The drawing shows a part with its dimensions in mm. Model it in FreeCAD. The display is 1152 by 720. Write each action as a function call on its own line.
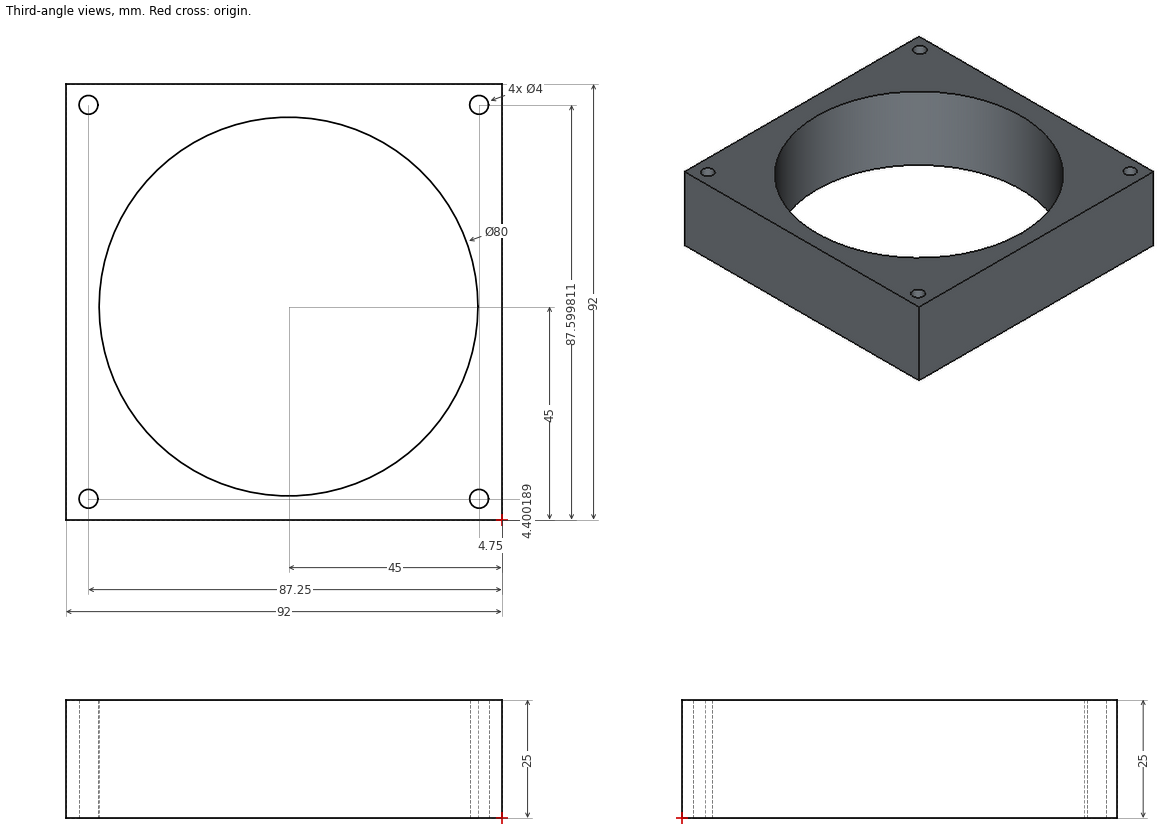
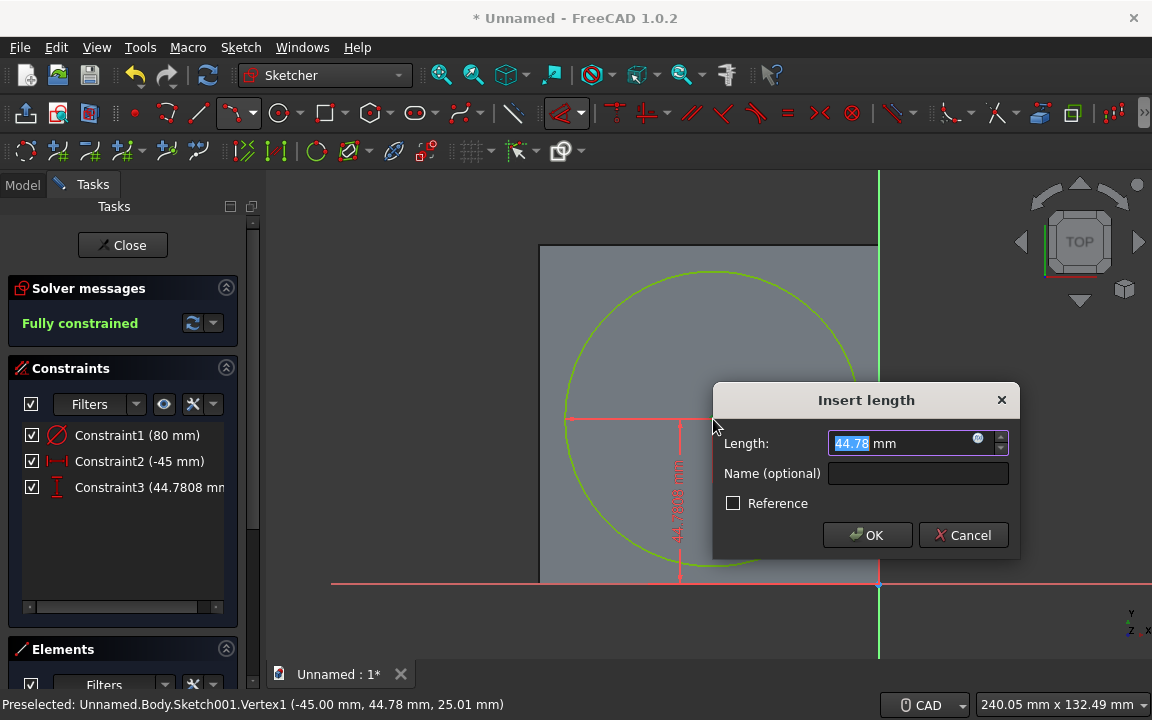
text(45)
key(Return)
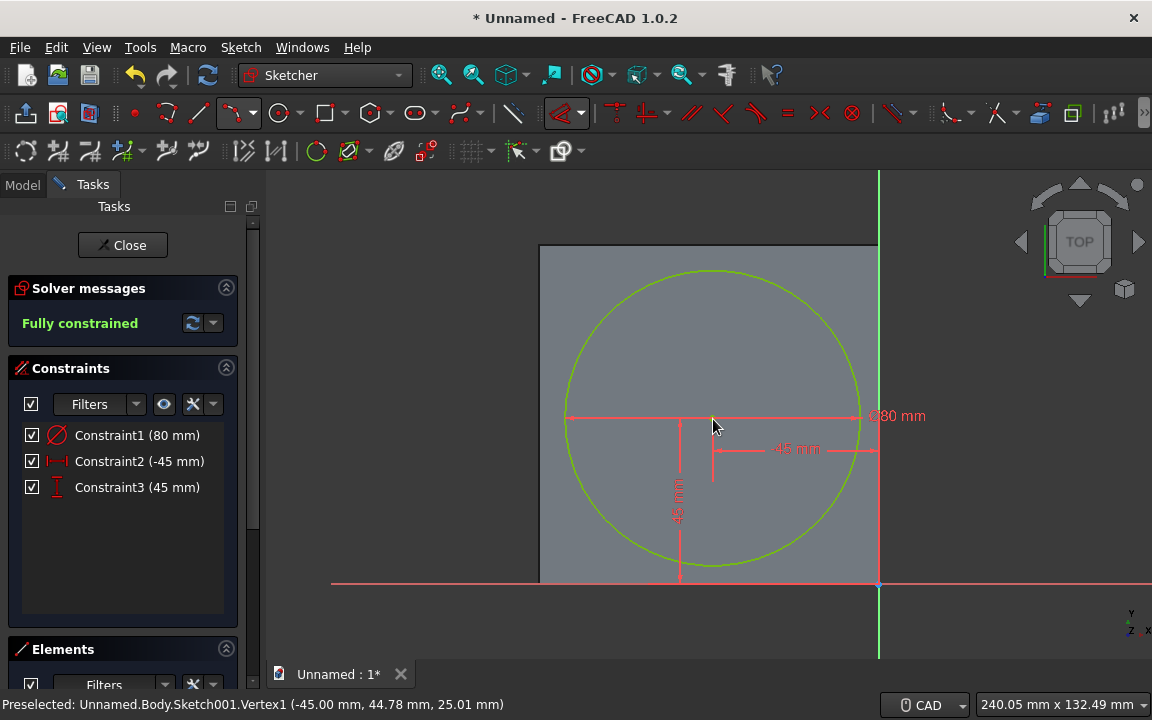
click(123, 245)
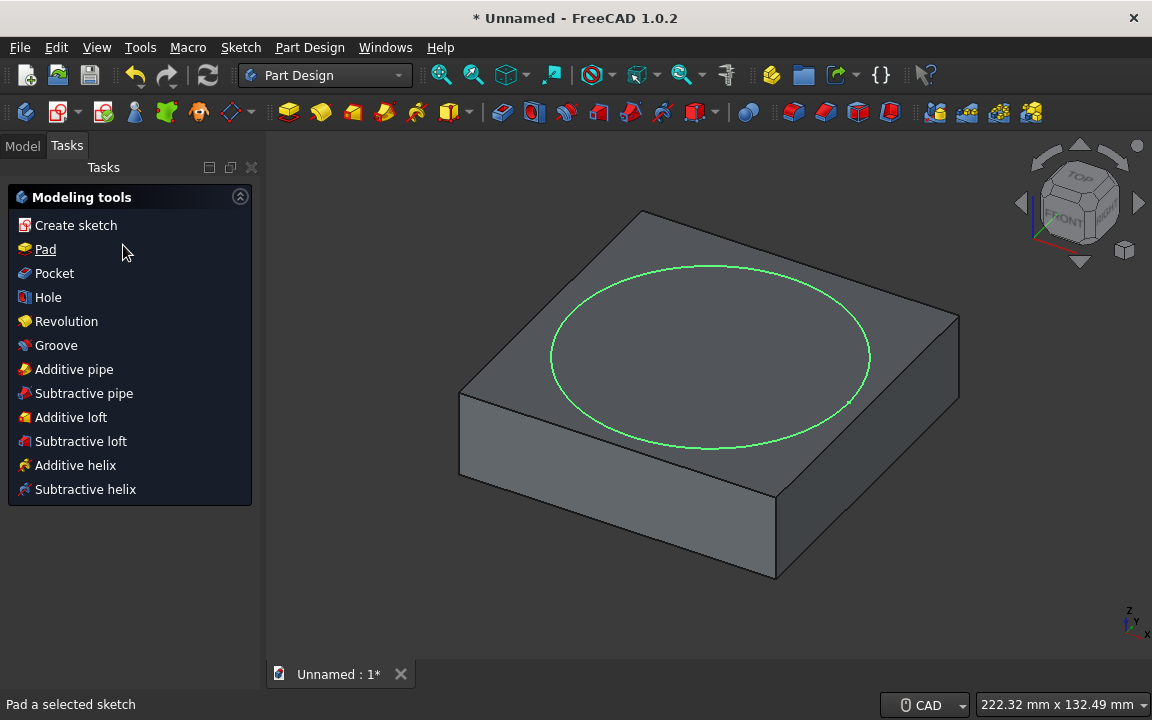
click(504, 112)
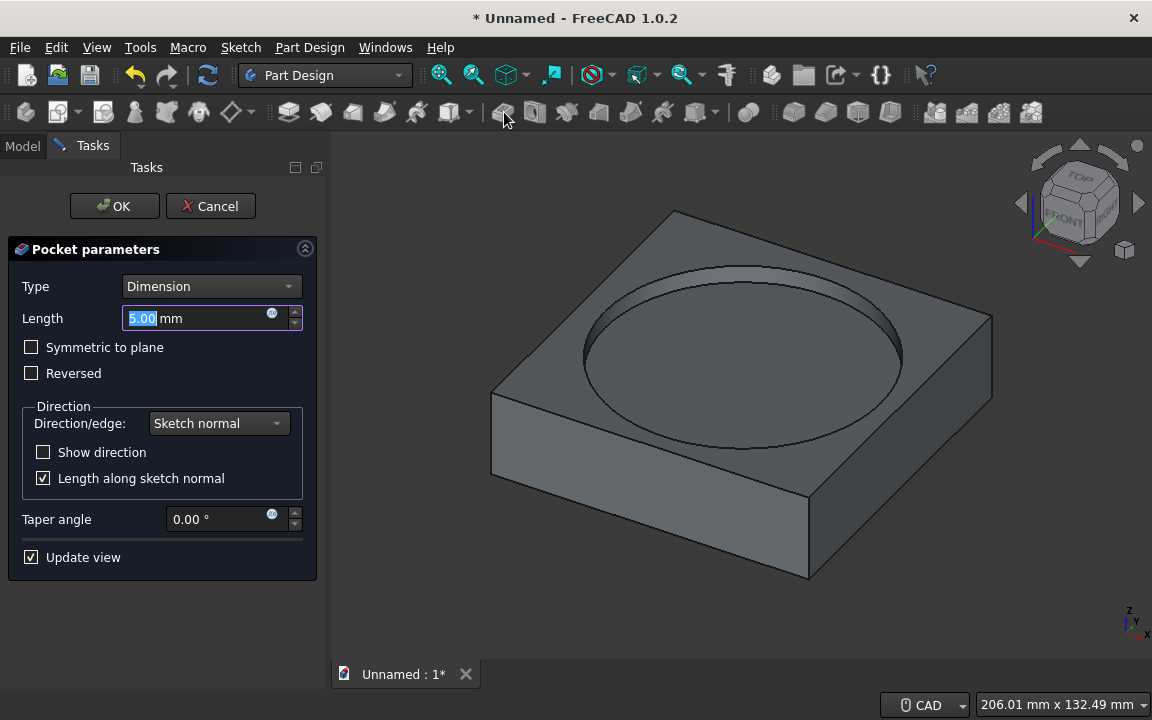
text(25)
key(Tab)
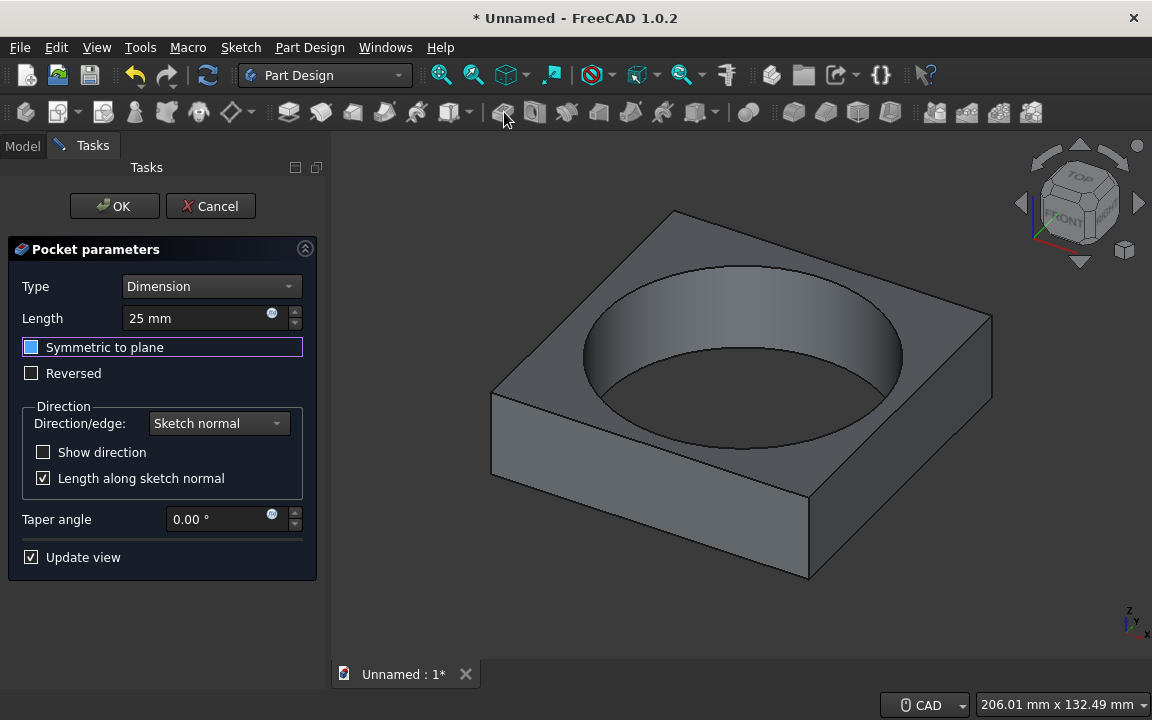
click(115, 206)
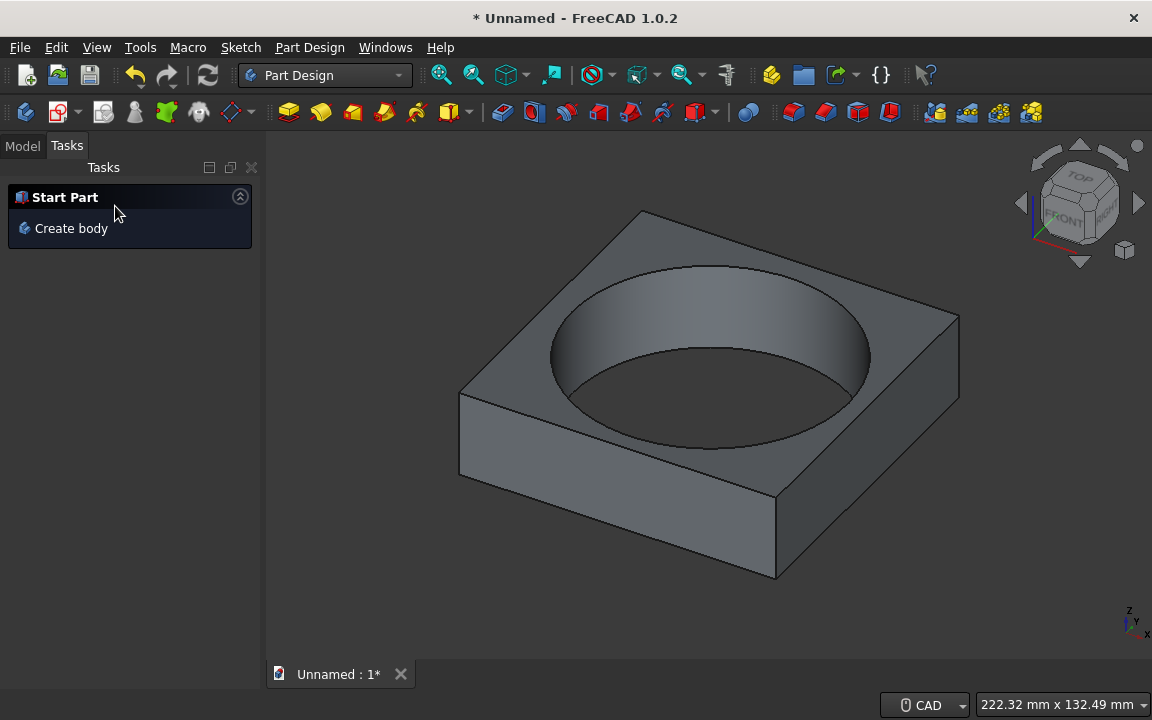
click(924, 320)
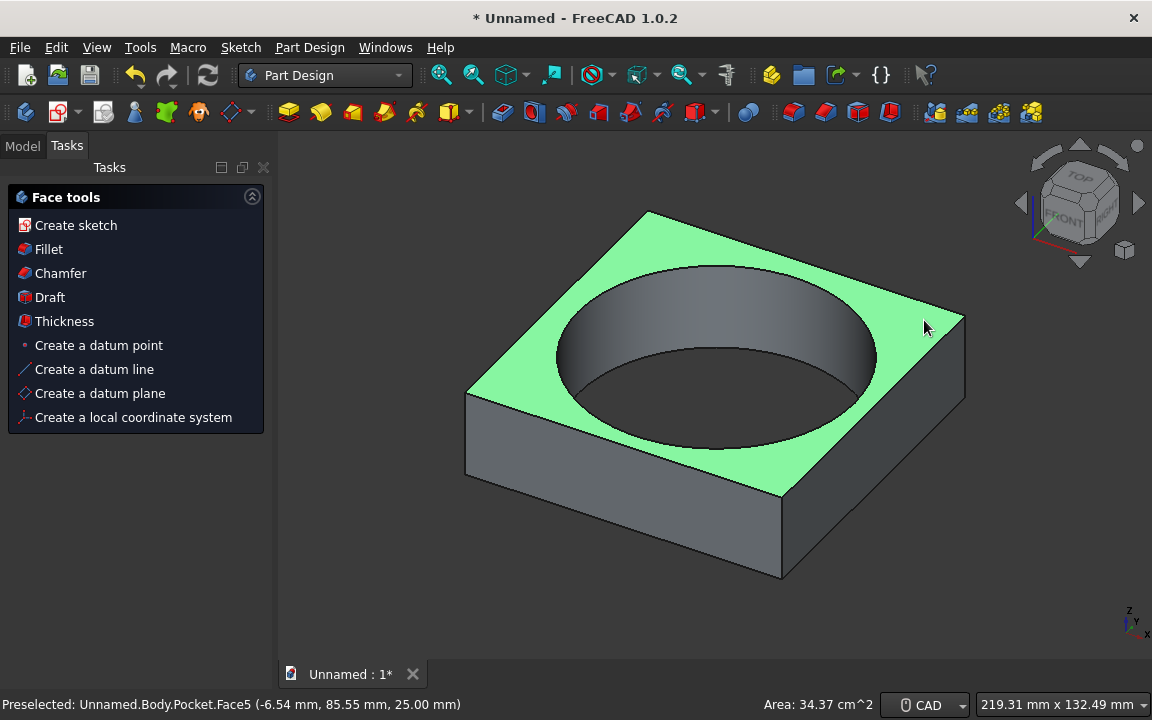
click(58, 112)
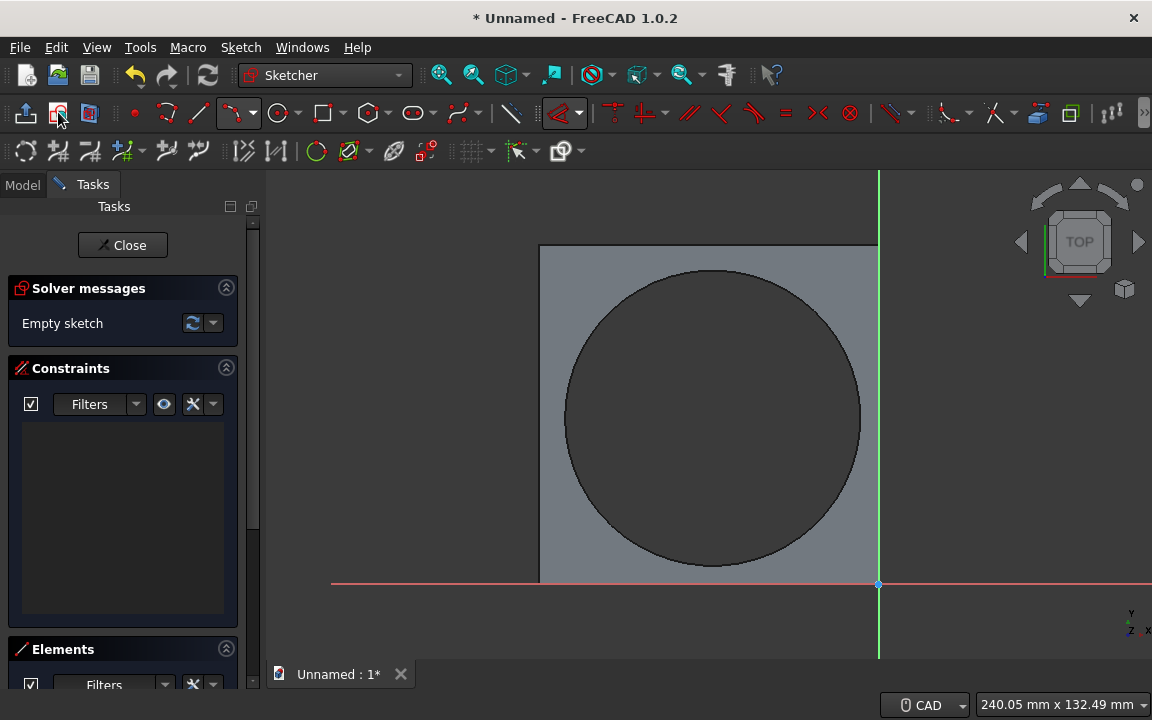
key(g)
key(c)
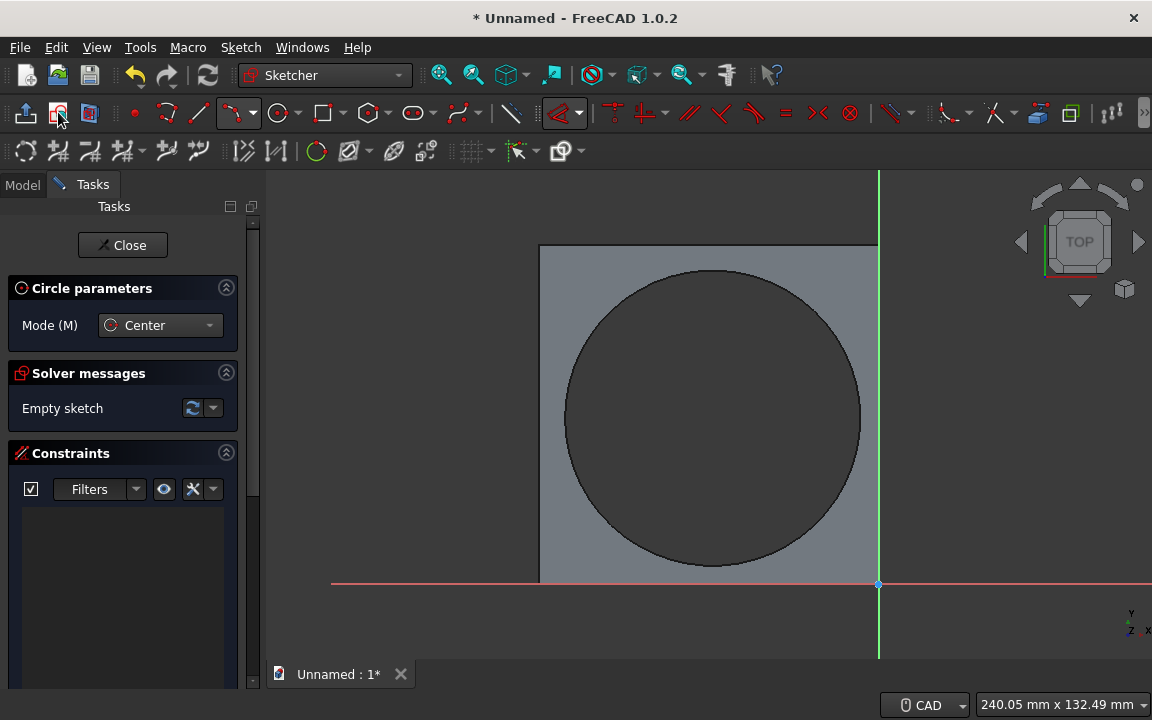
scroll(861, 261, up, 6)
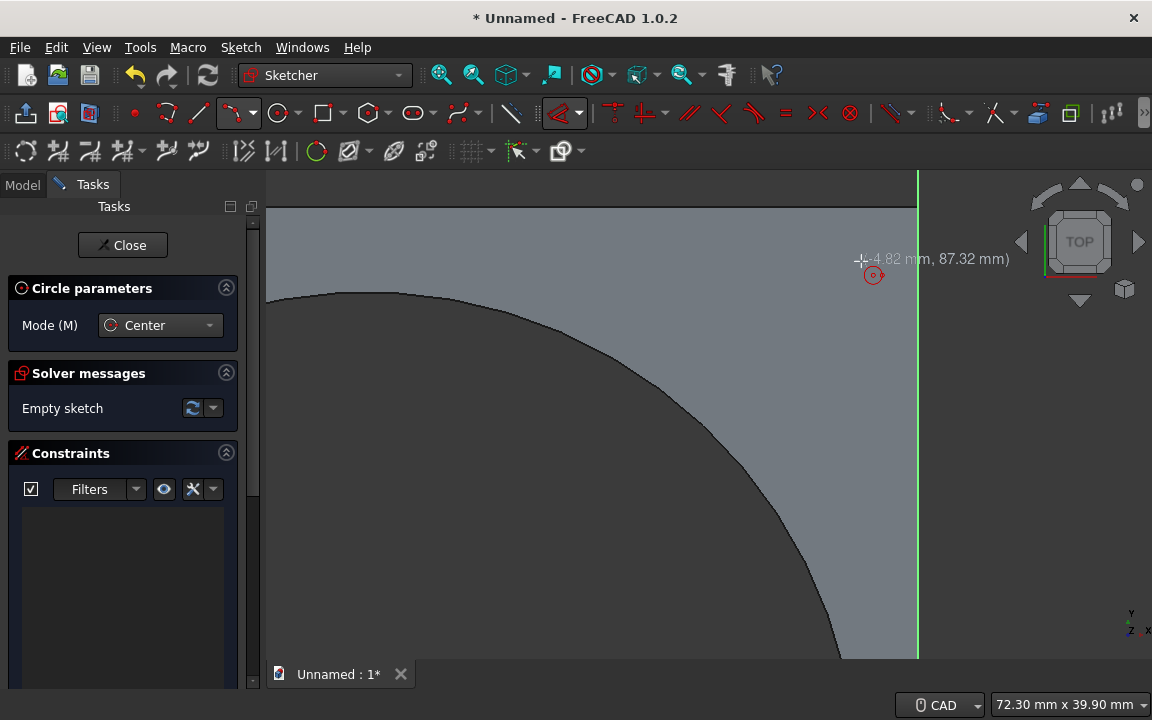
click(860, 260)
move(878, 243)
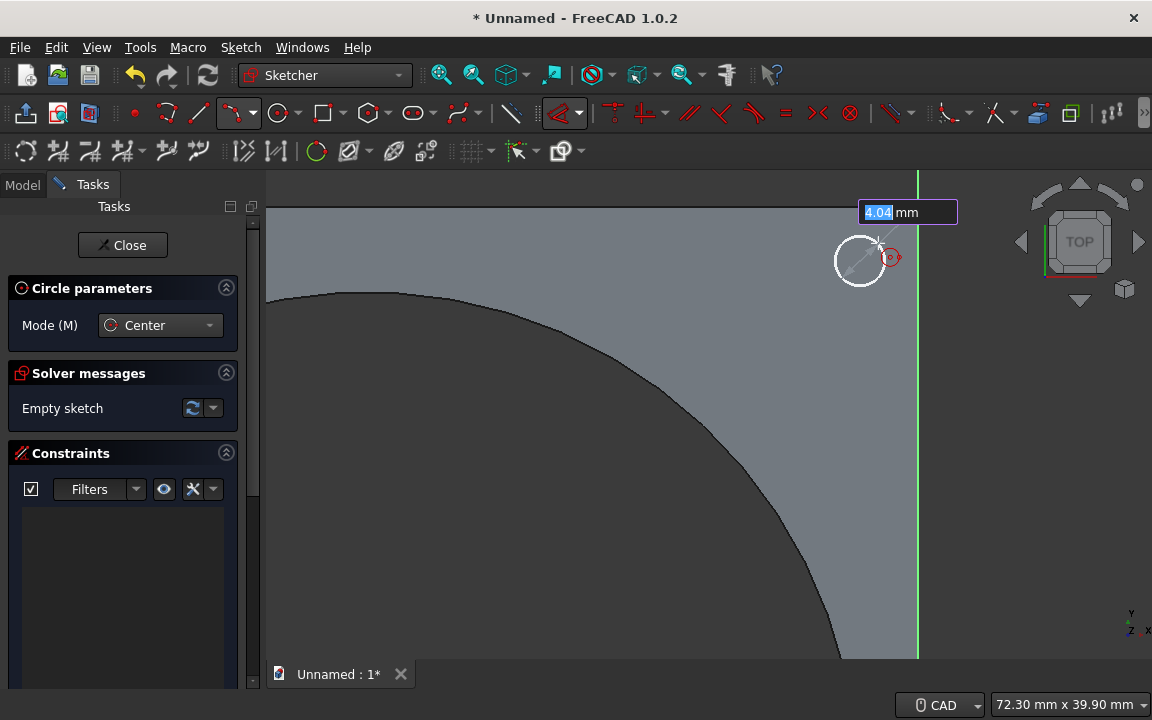
text(4)
key(Return)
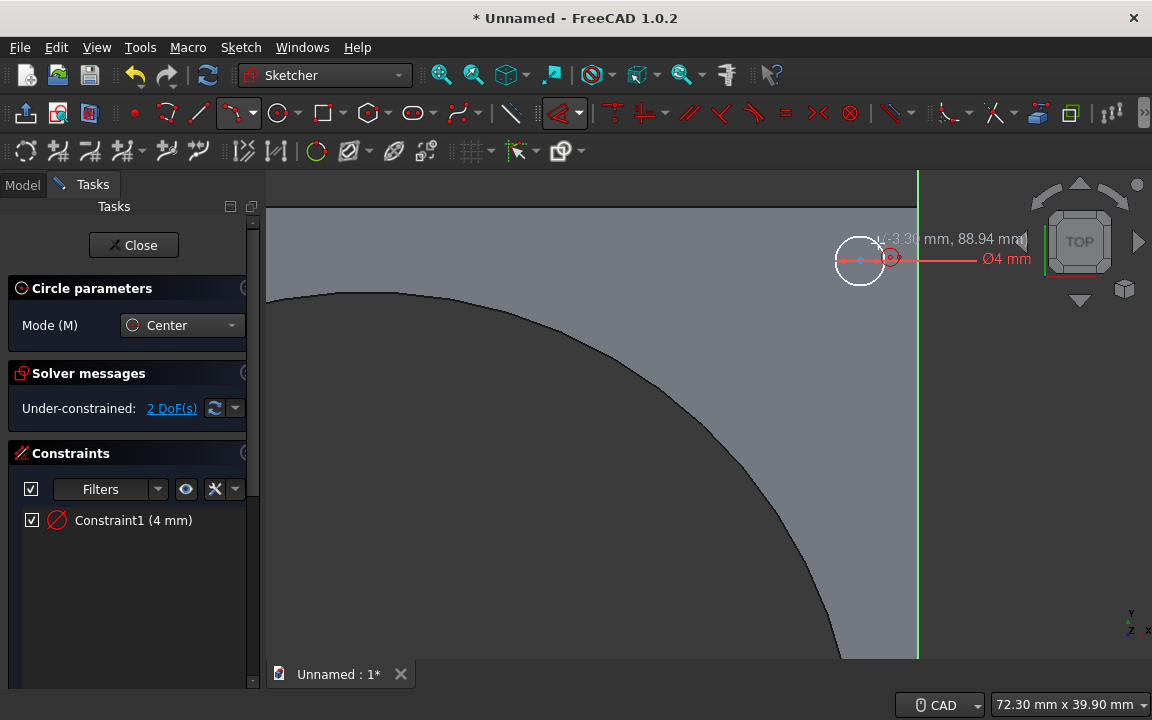
scroll(756, 255, down, 6)